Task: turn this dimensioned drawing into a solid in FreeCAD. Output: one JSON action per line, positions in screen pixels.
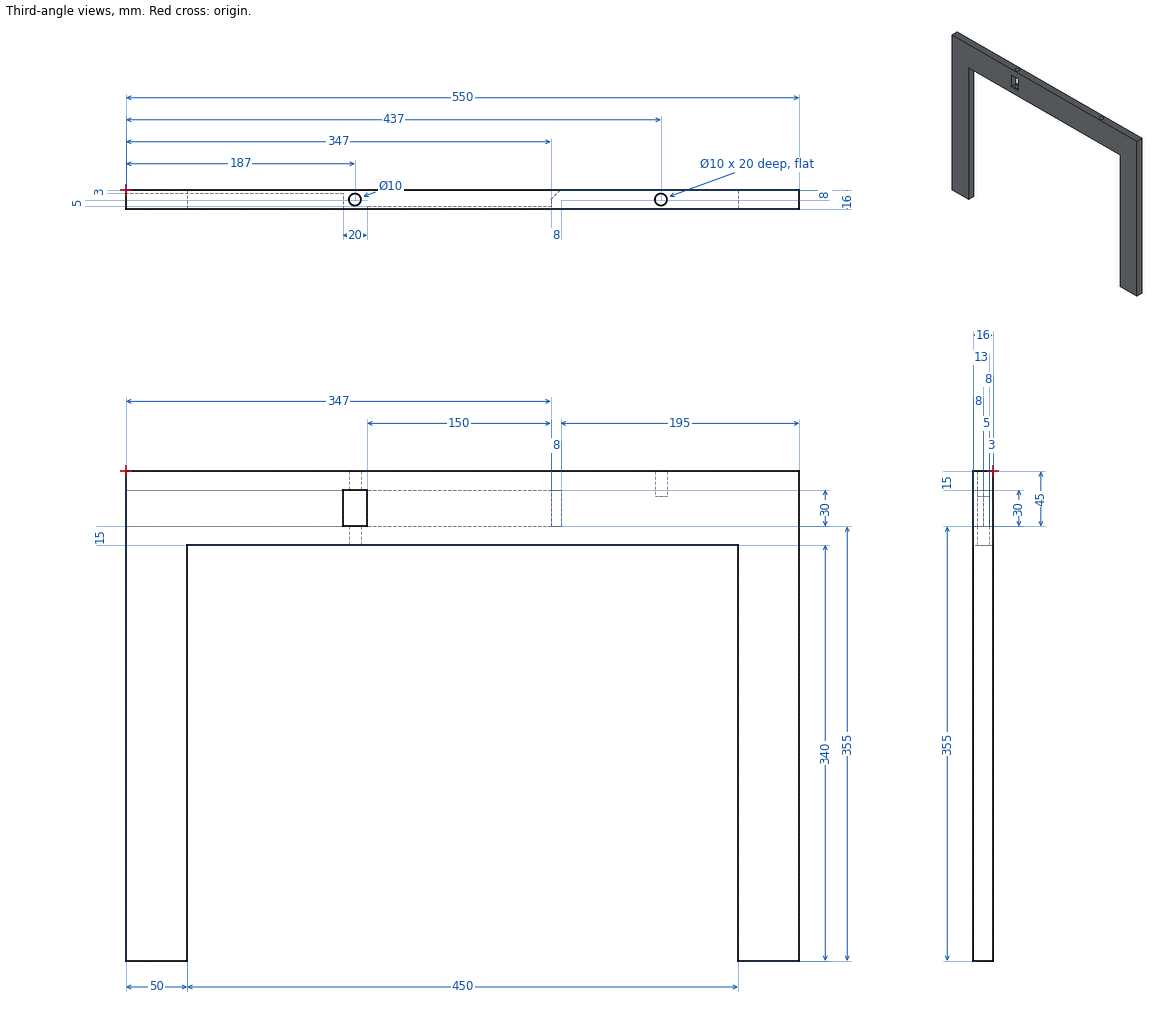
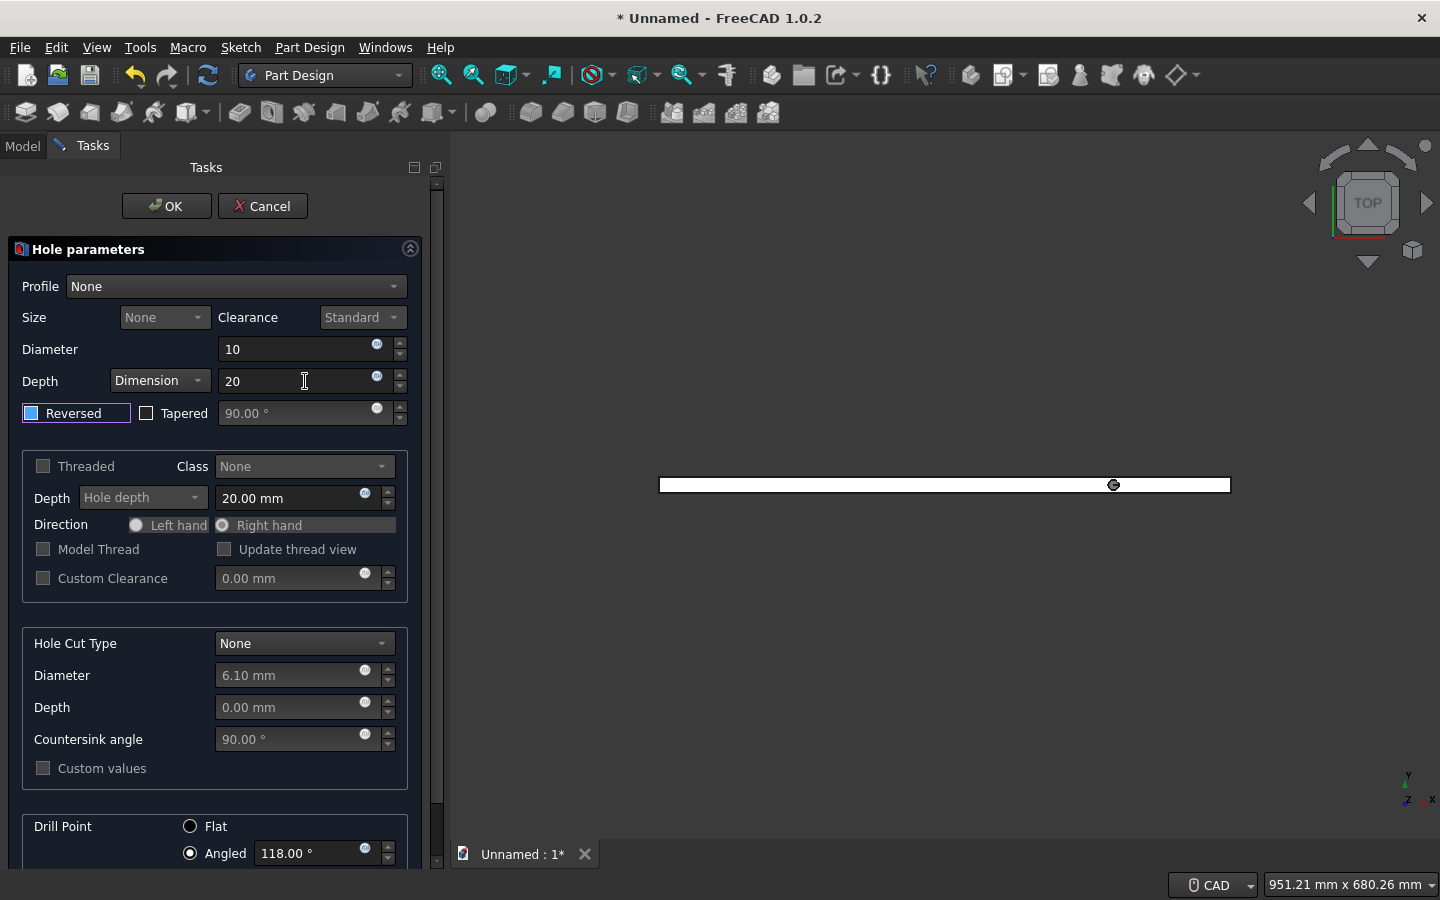
{"action": "left_click", "coordinate": [191, 826]}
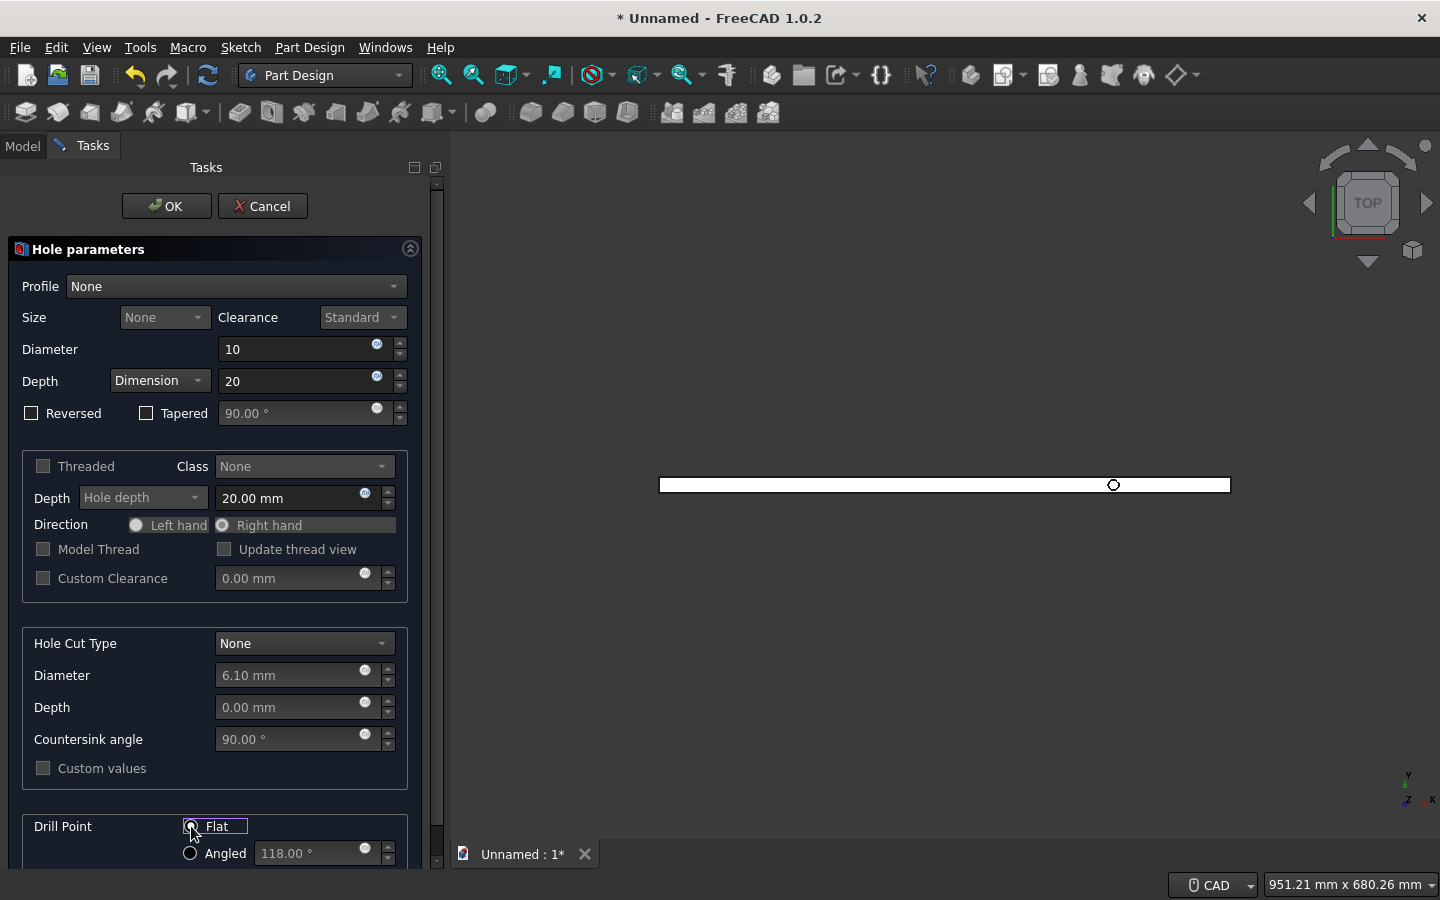
{"action": "left_click", "coordinate": [167, 206]}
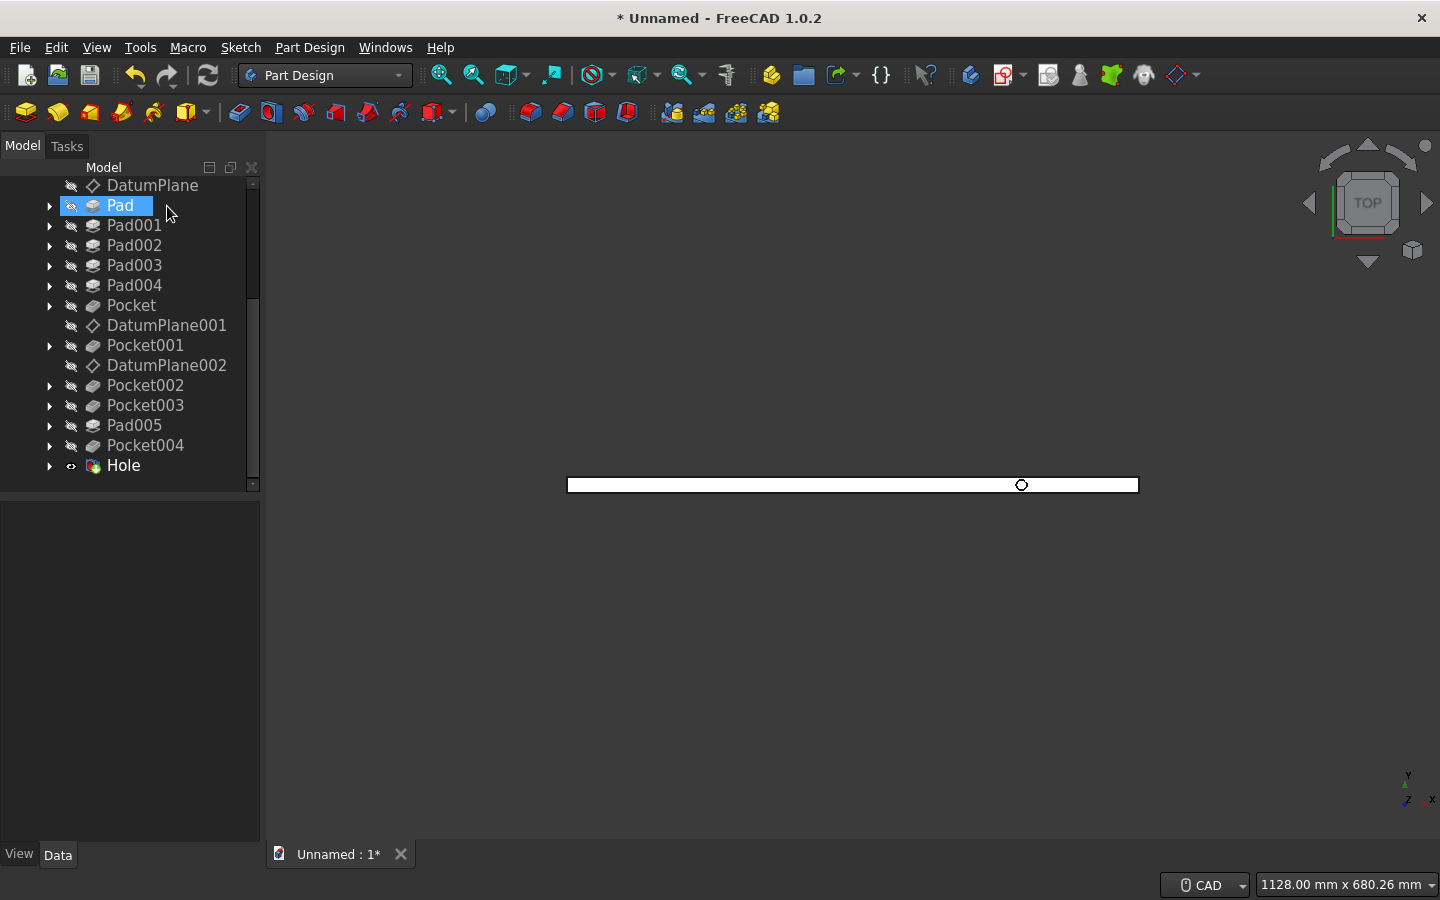
{"action": "left_click", "coordinate": [1098, 484]}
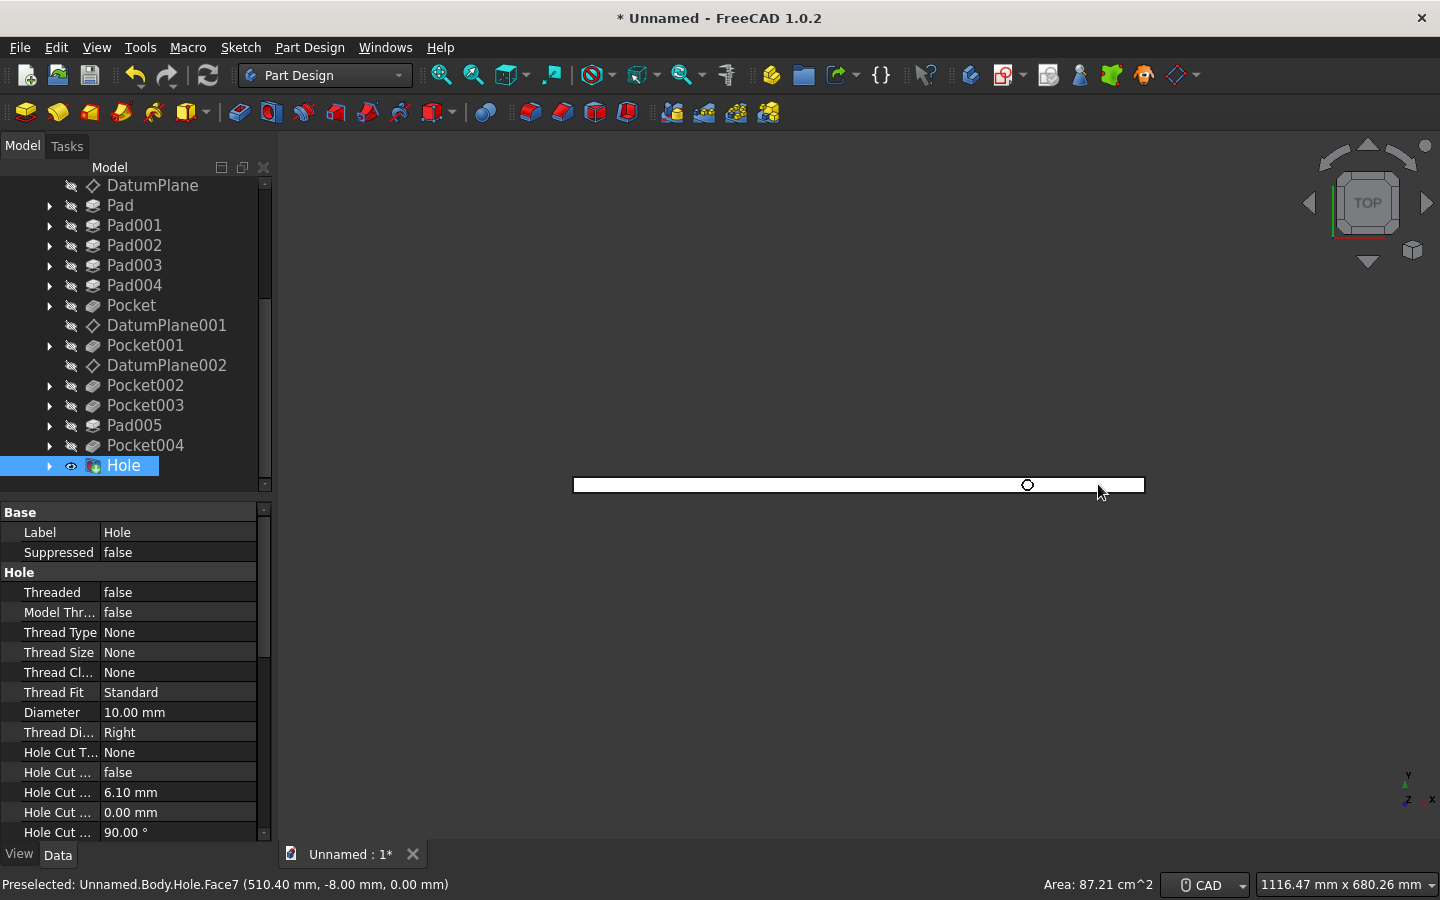
{"action": "left_click", "coordinate": [1004, 76]}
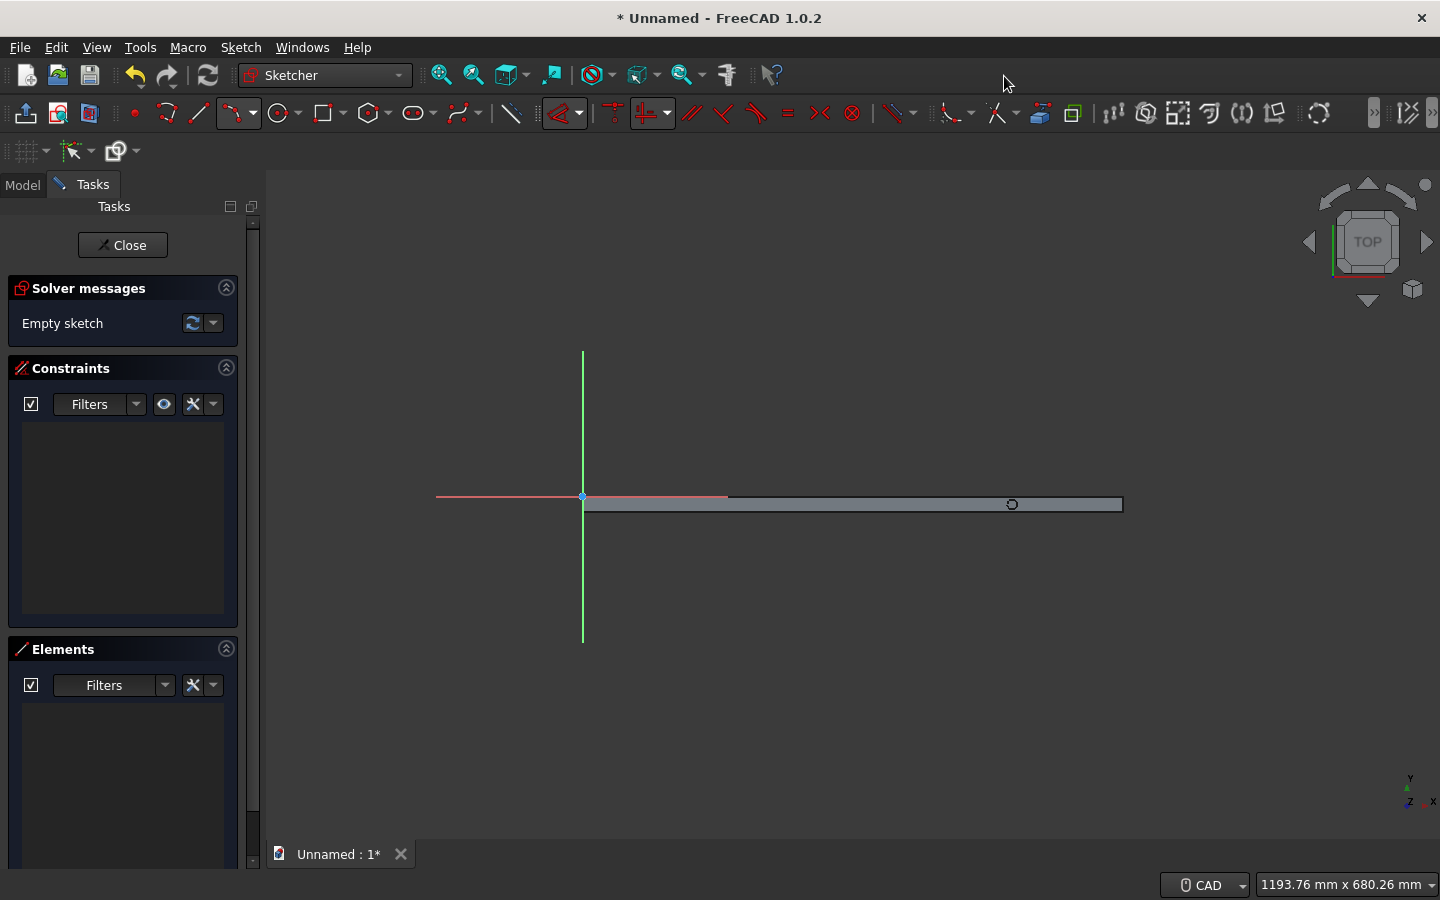
{"action": "scroll", "coordinate": [766, 504], "scroll_direction": "up", "scroll_amount": 15}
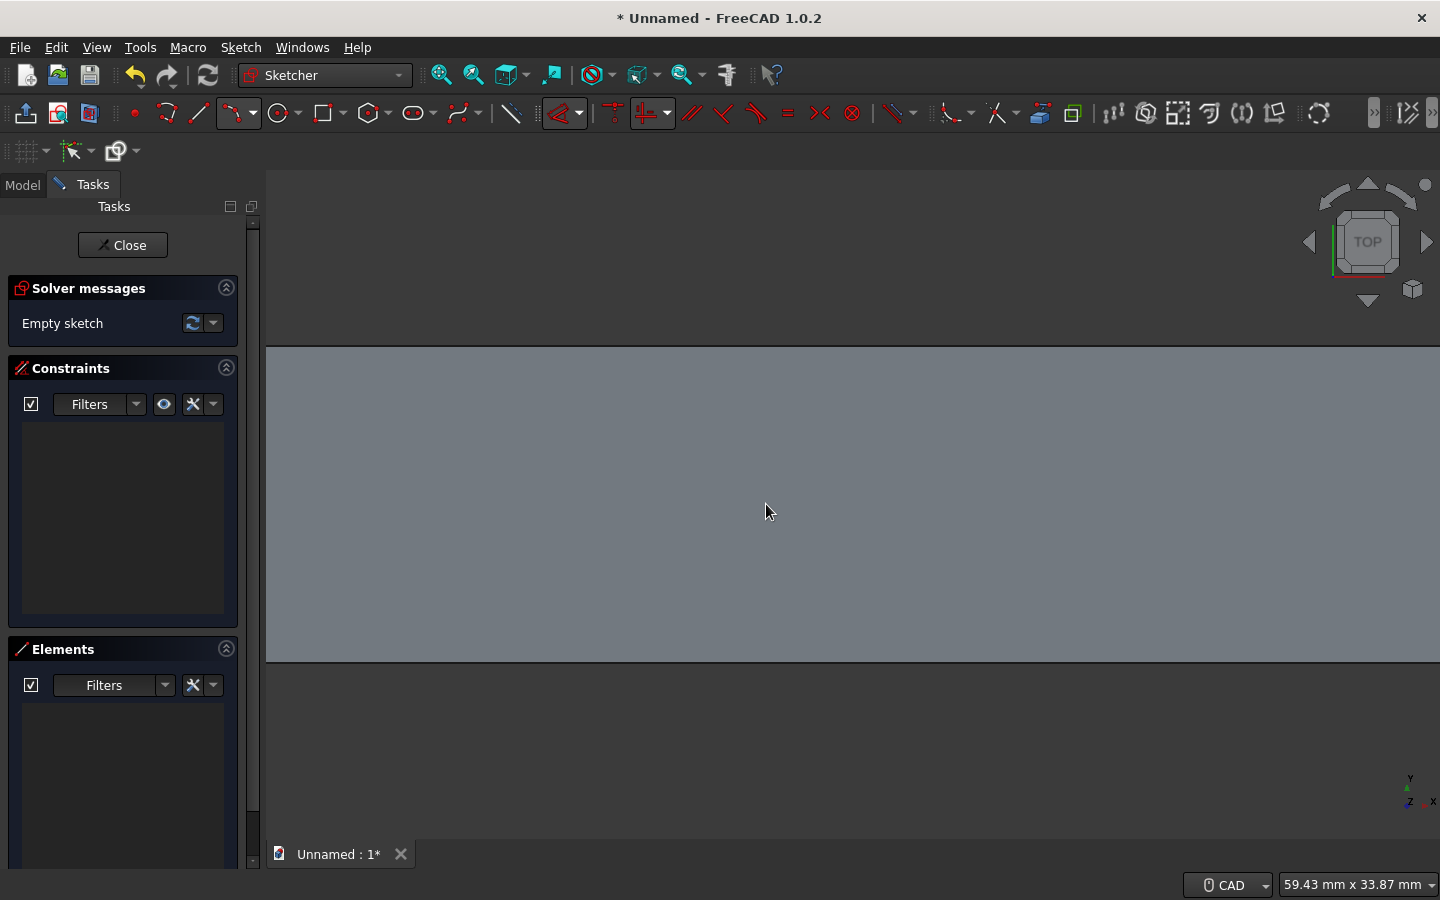
{"action": "scroll", "coordinate": [753, 504], "scroll_direction": "up", "scroll_amount": 4}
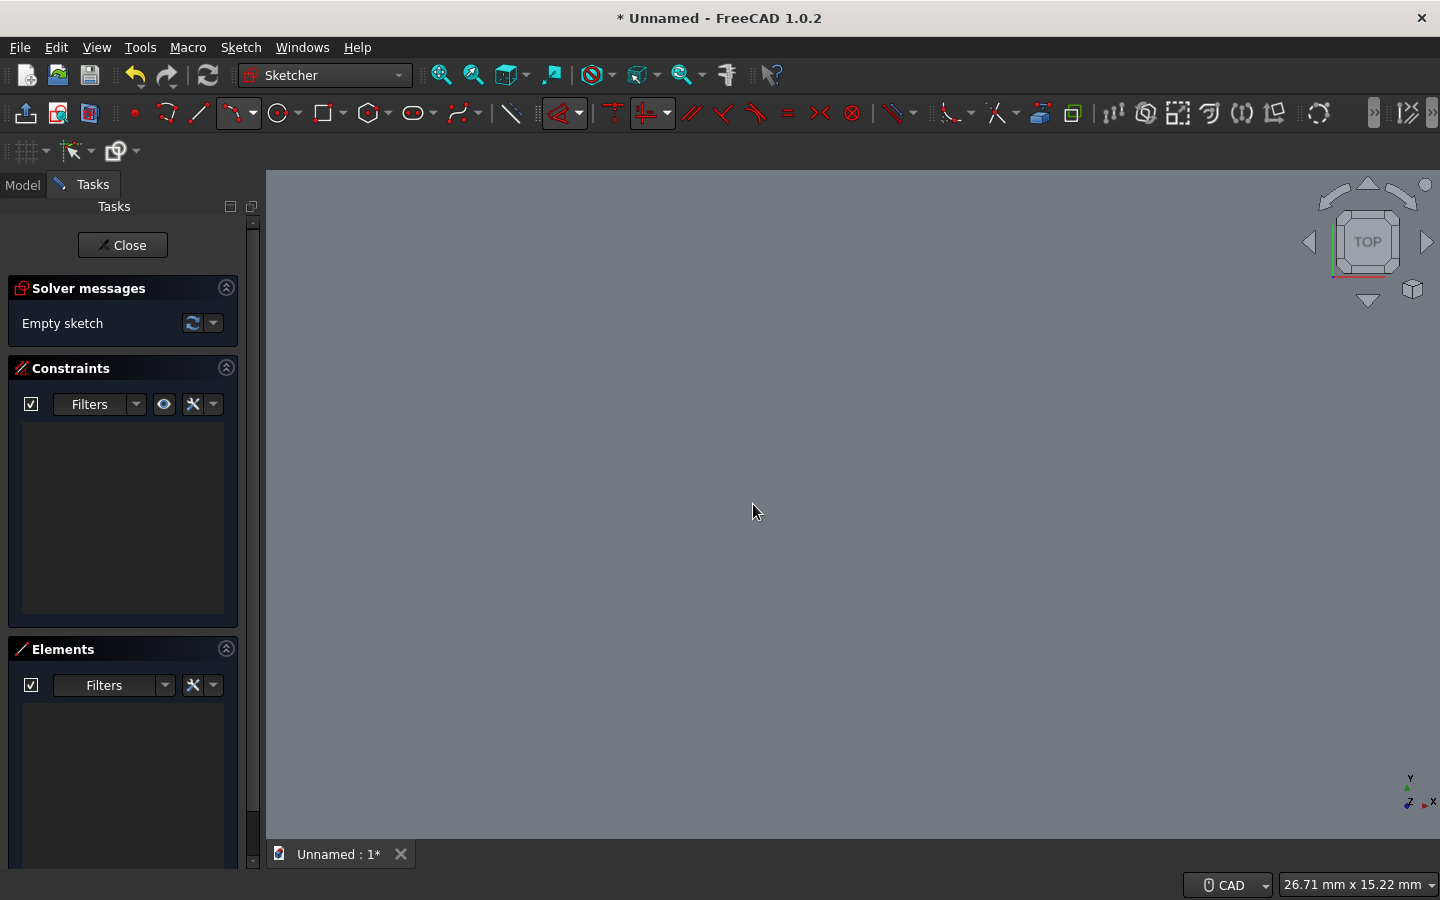
{"action": "left_click", "coordinate": [278, 114]}